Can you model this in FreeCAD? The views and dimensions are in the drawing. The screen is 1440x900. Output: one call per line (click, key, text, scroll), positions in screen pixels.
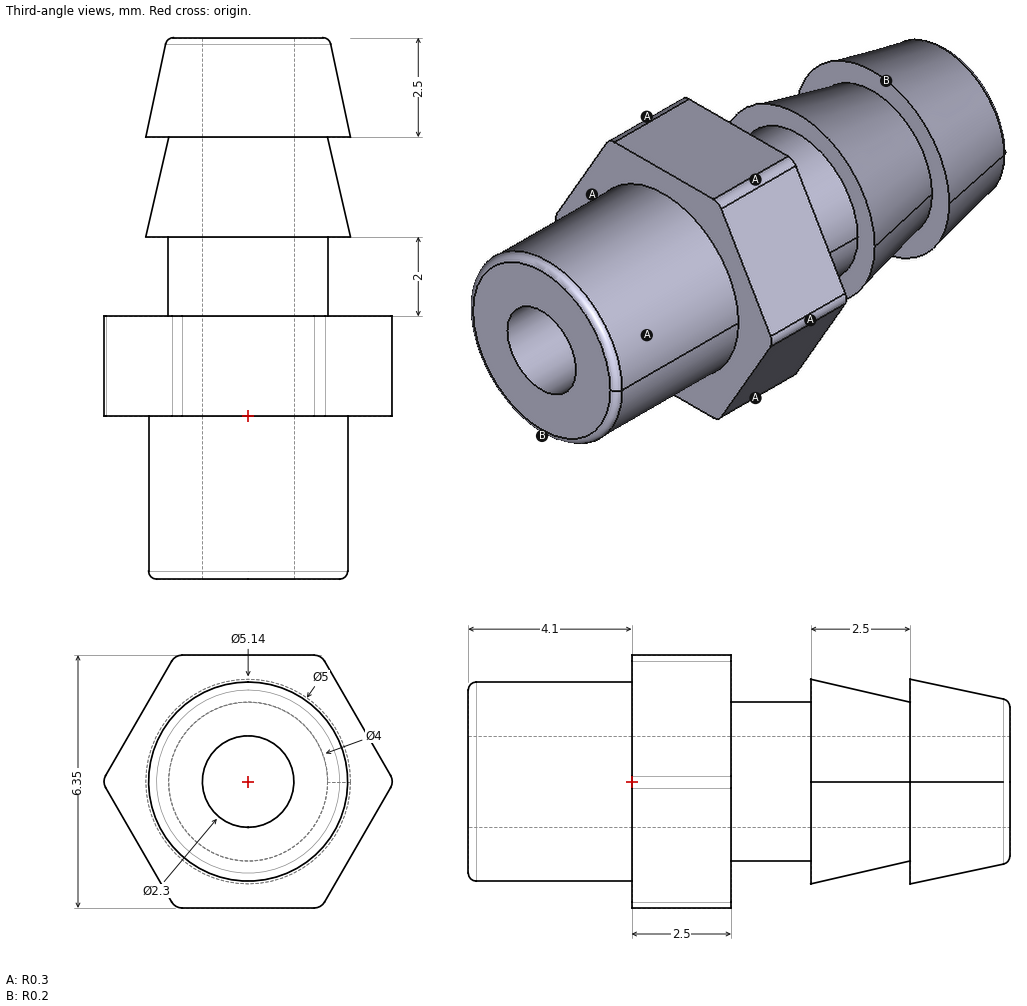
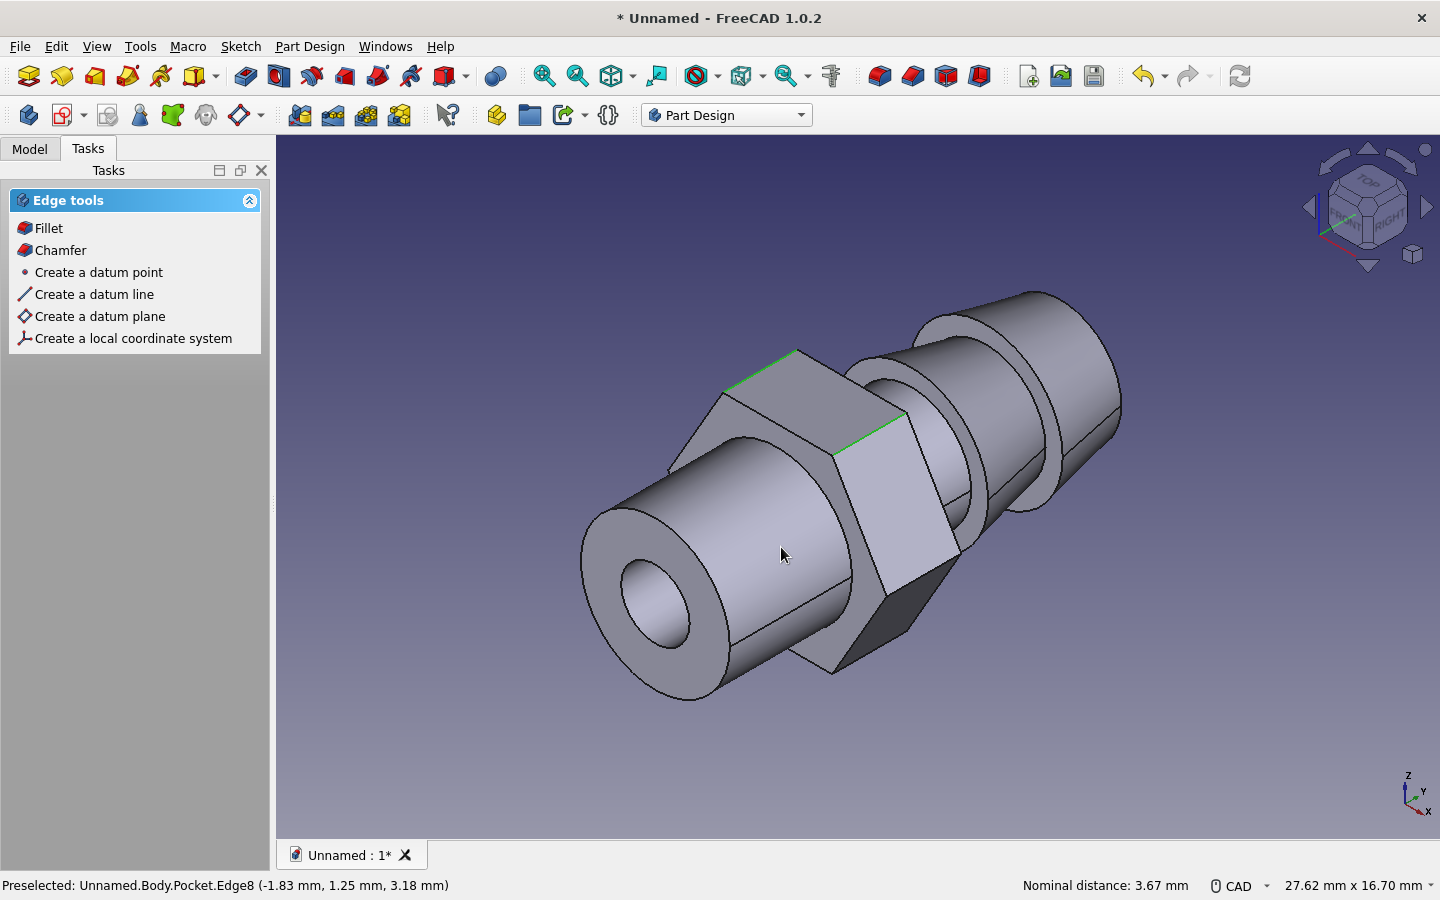
key(1)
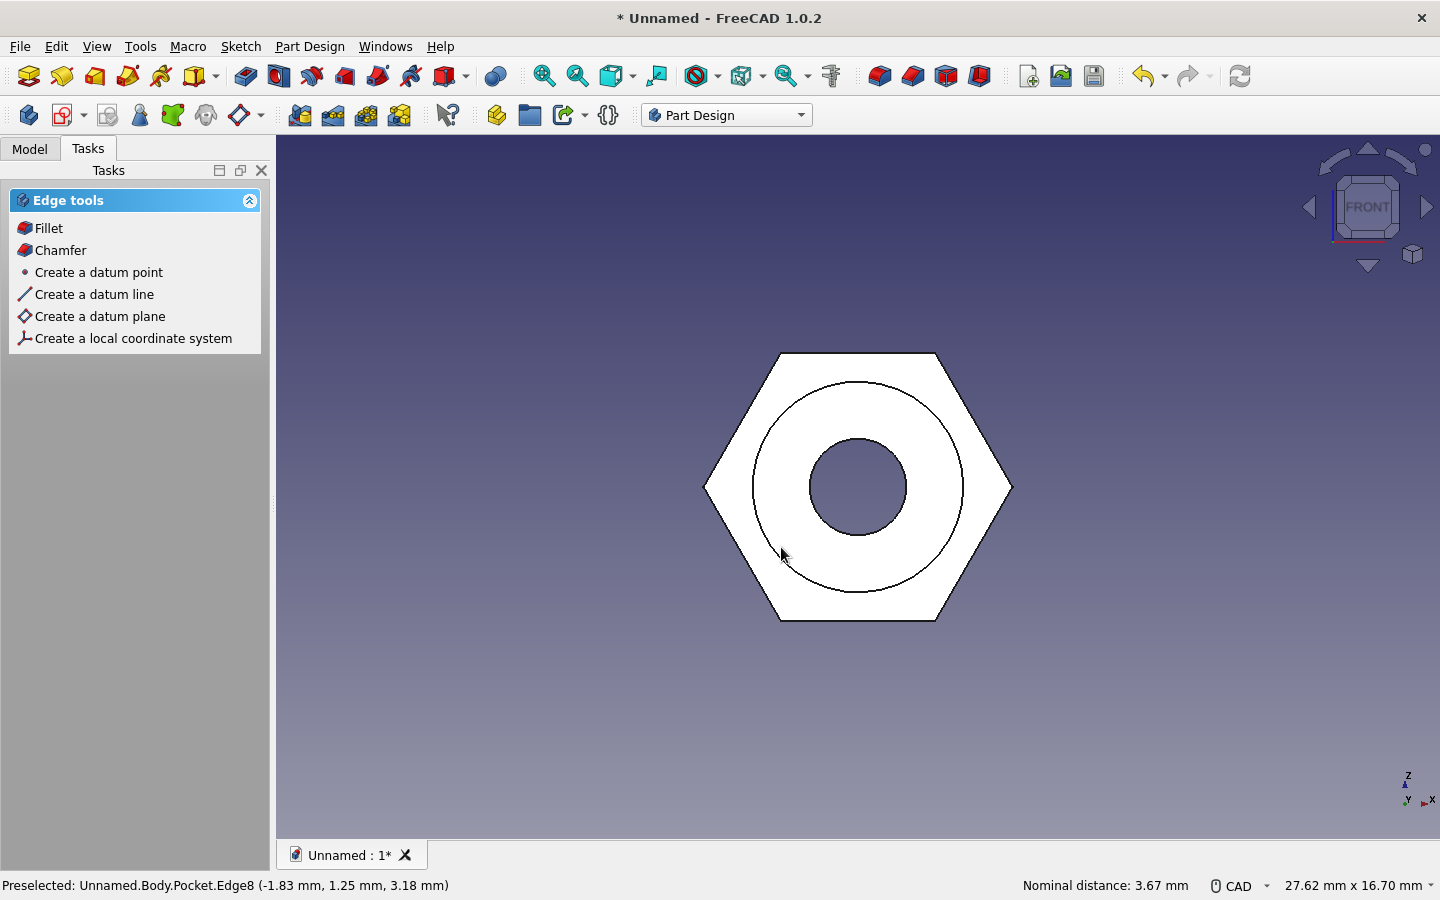
click(545, 76)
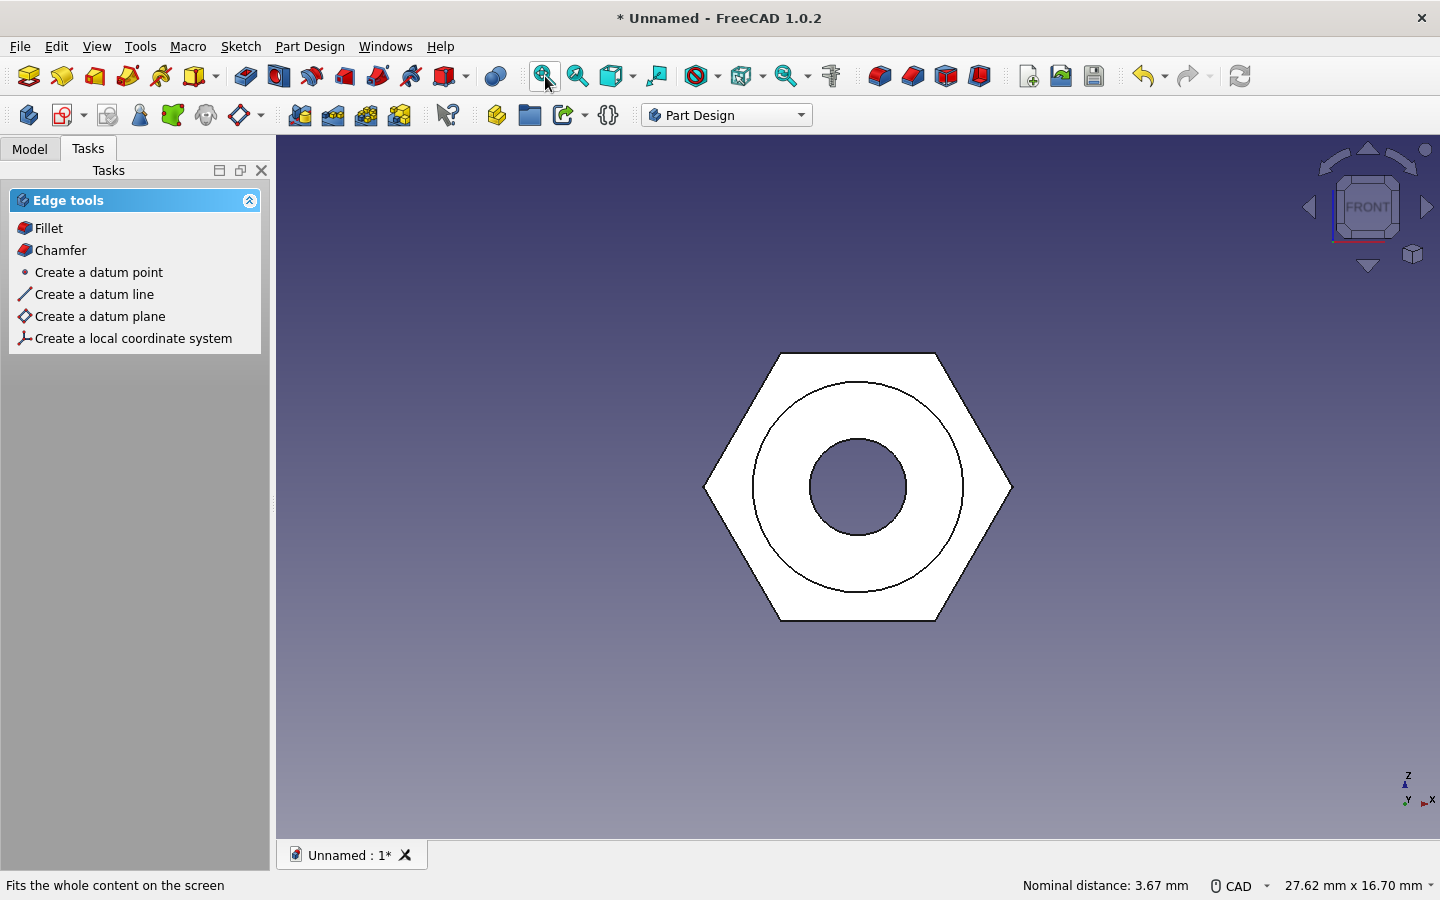
key(3)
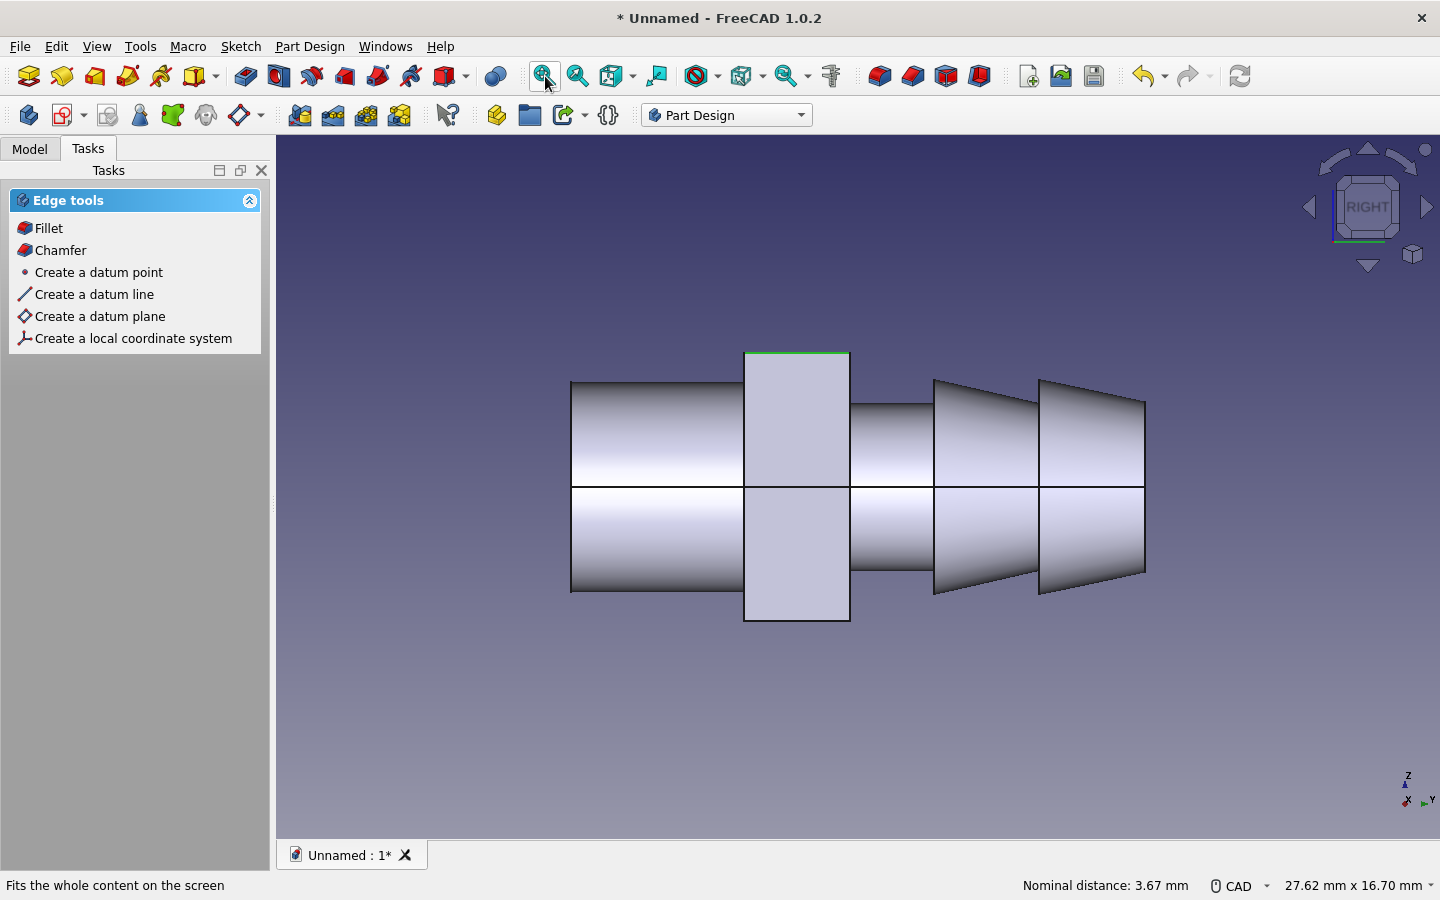
click(797, 486, ctrl)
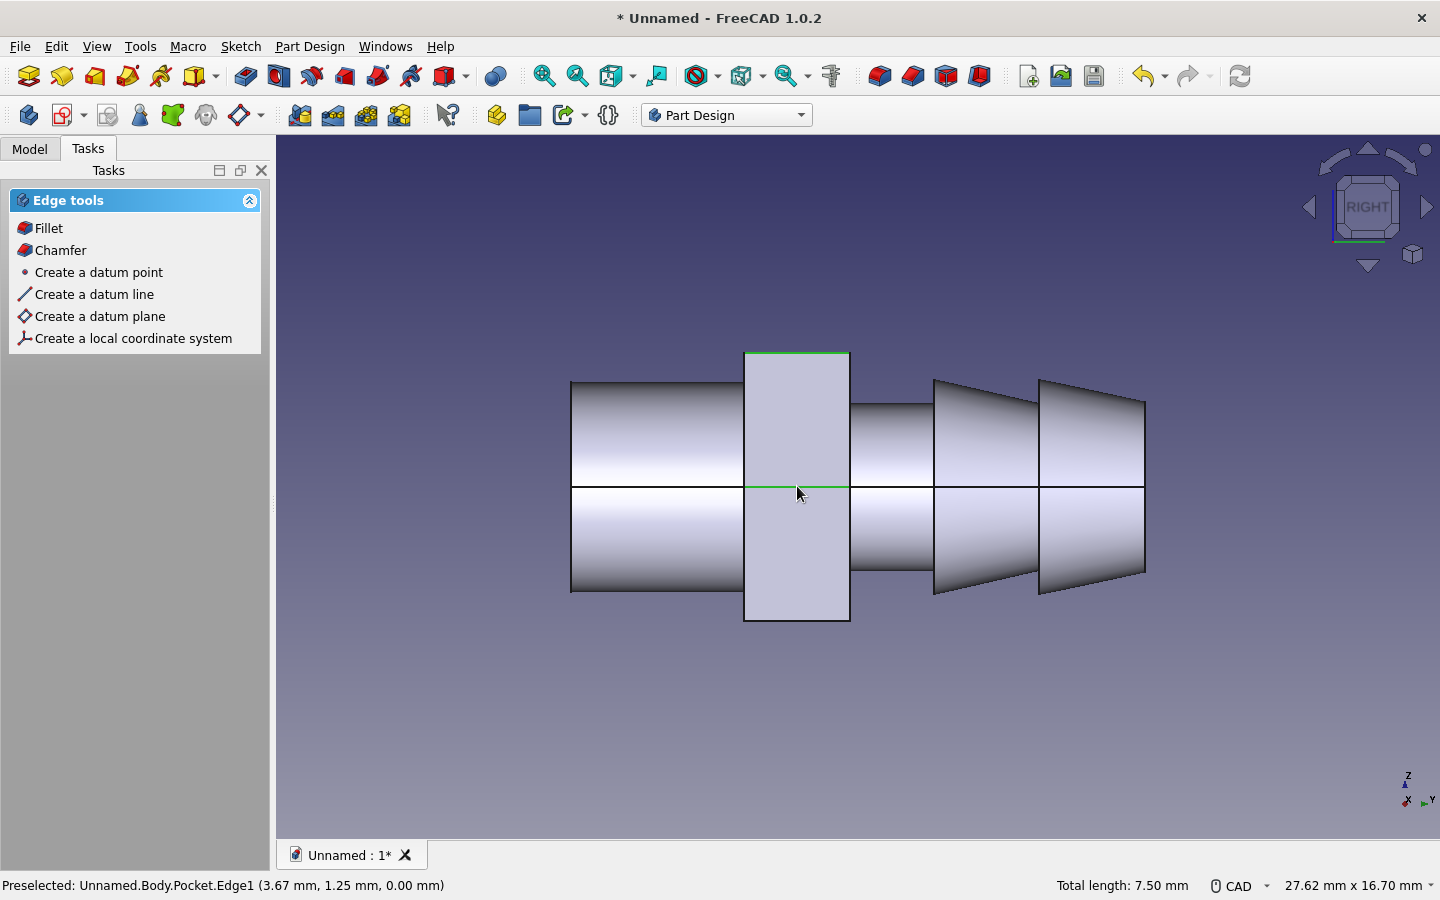
key(5)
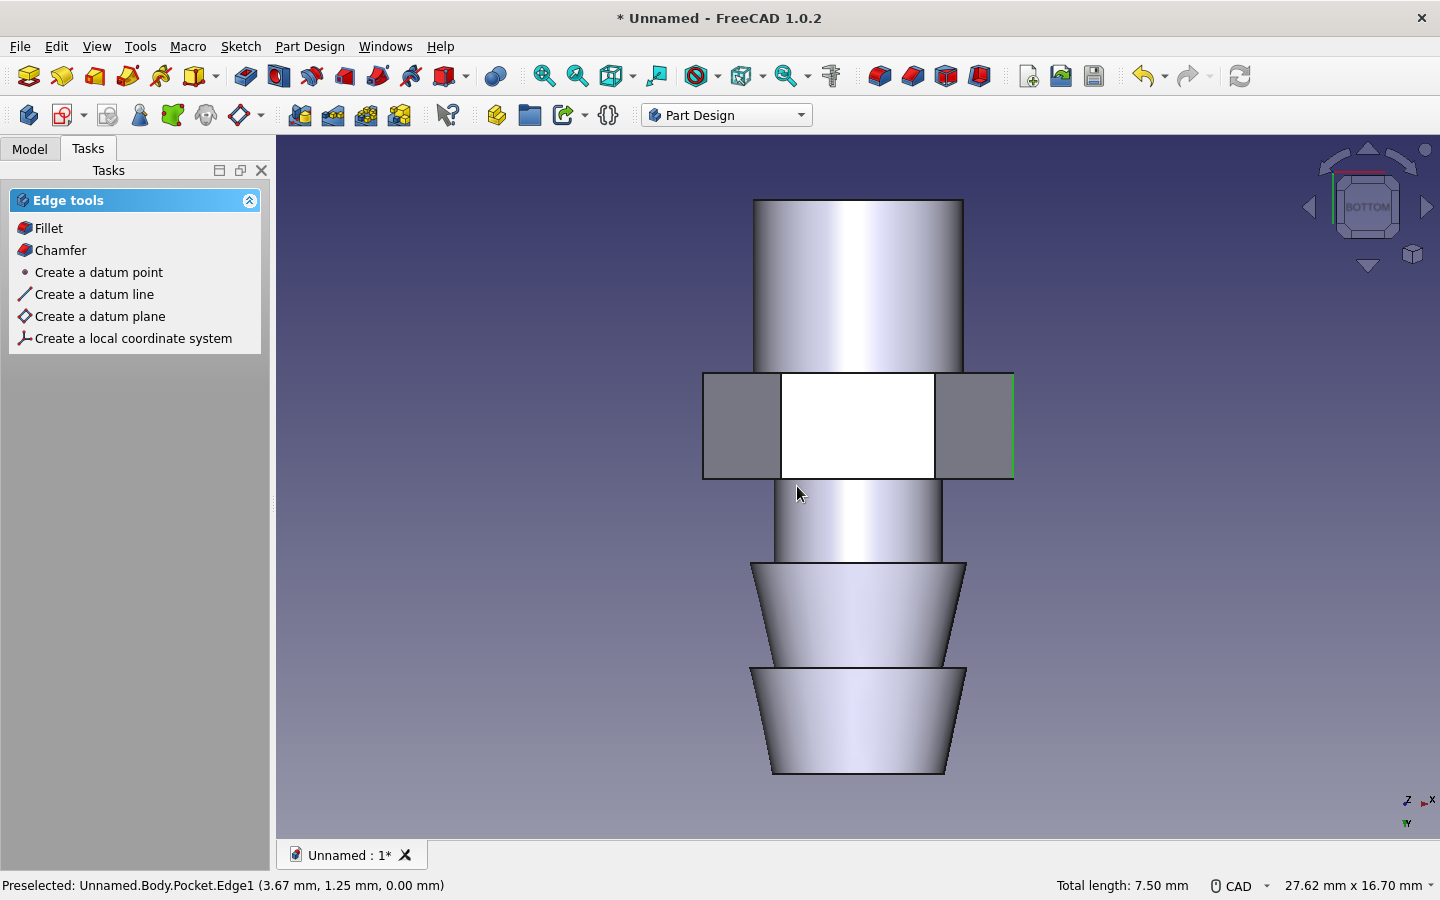
click(781, 425, ctrl)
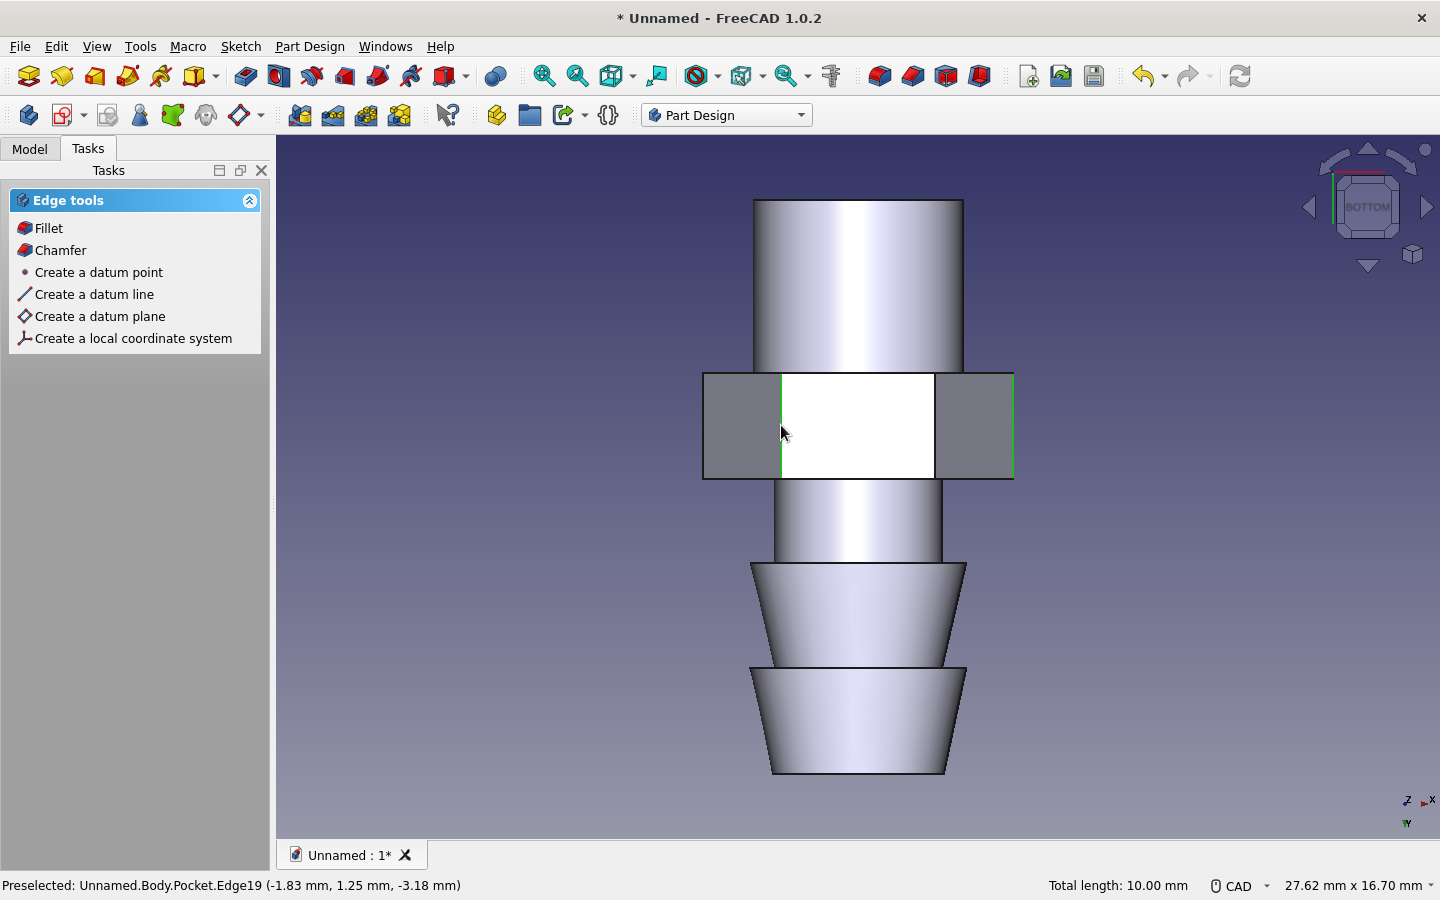
click(935, 425, ctrl)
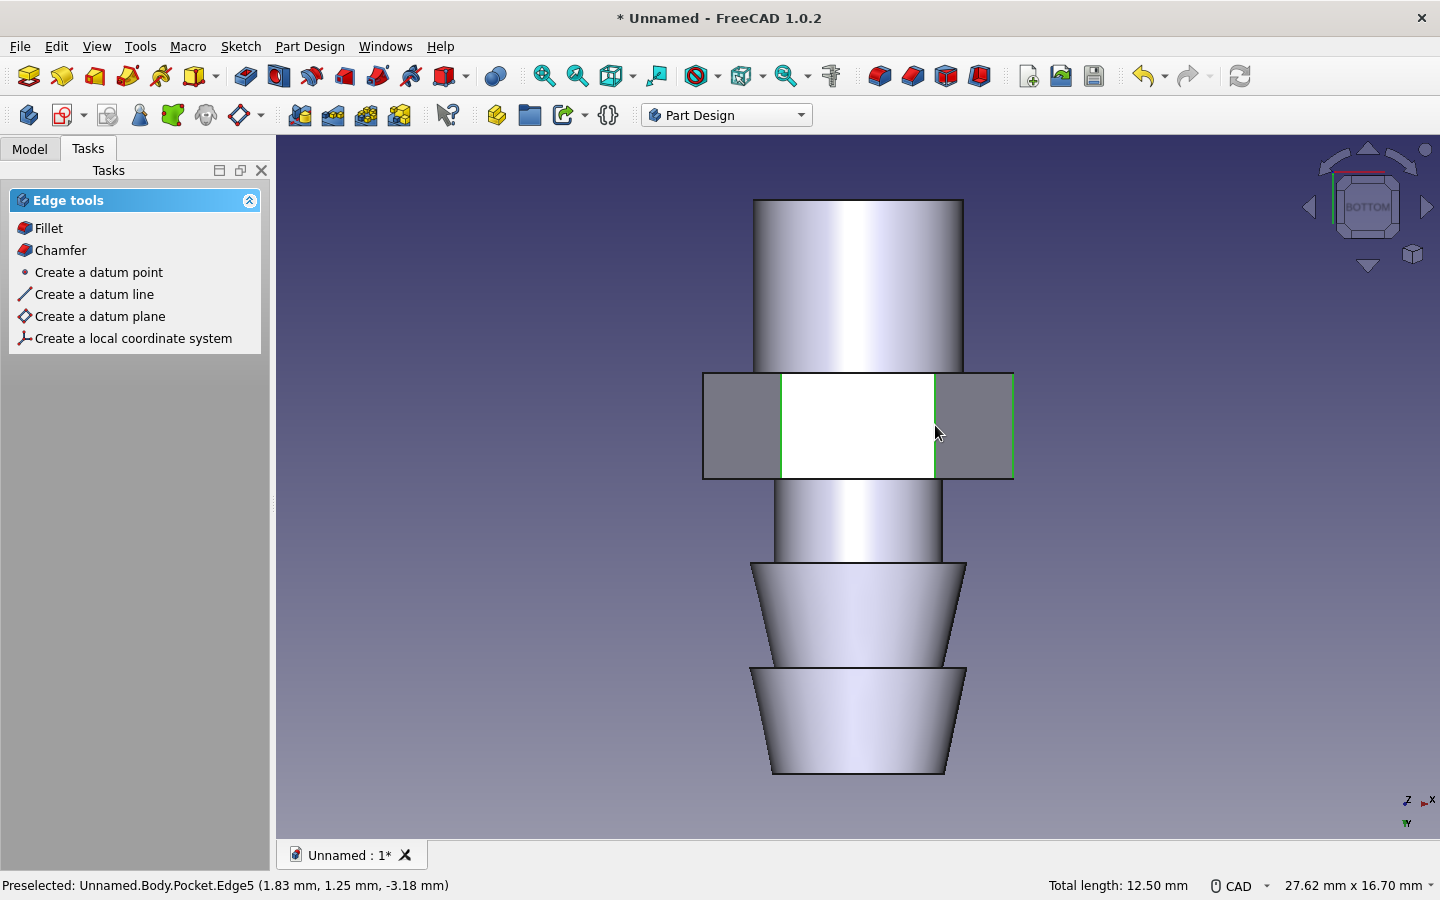
key(4)